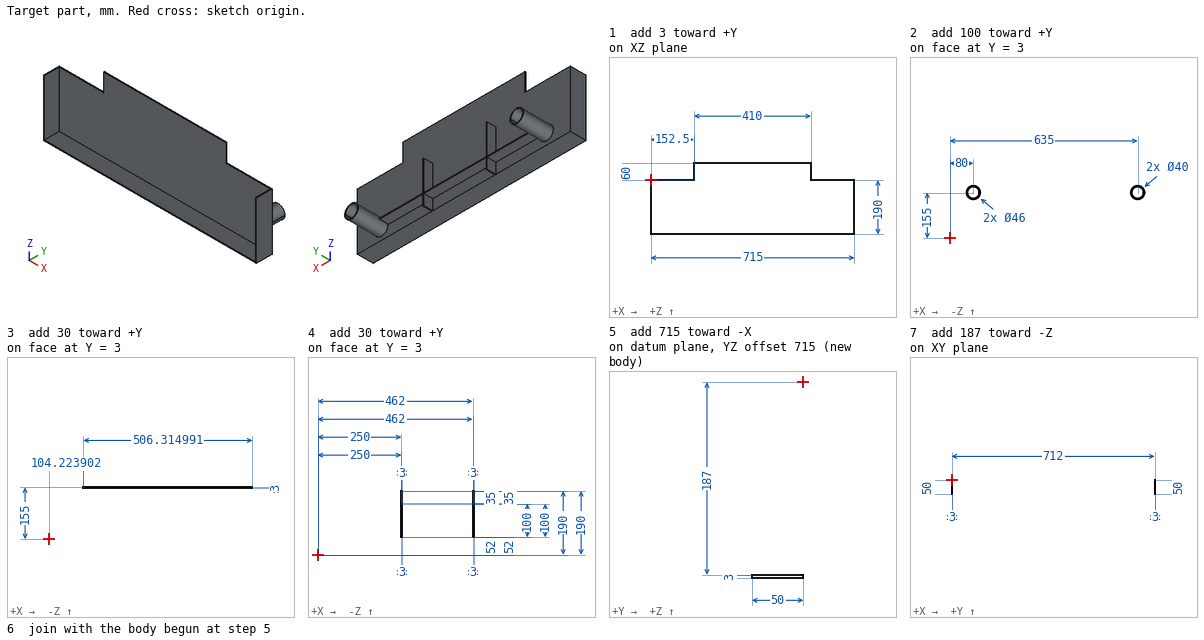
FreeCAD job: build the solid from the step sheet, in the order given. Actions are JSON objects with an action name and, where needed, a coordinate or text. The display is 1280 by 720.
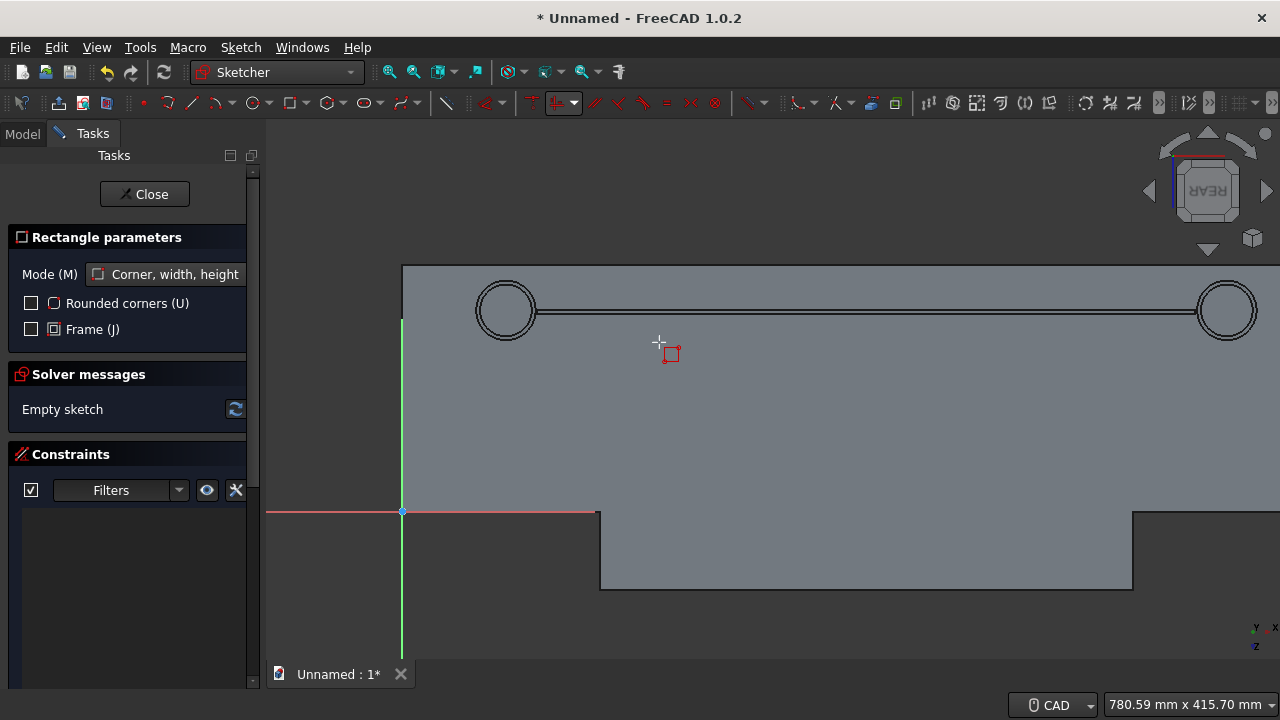
{"action": "scroll", "coordinate": [727, 265], "scroll_direction": "up", "scroll_amount": 8}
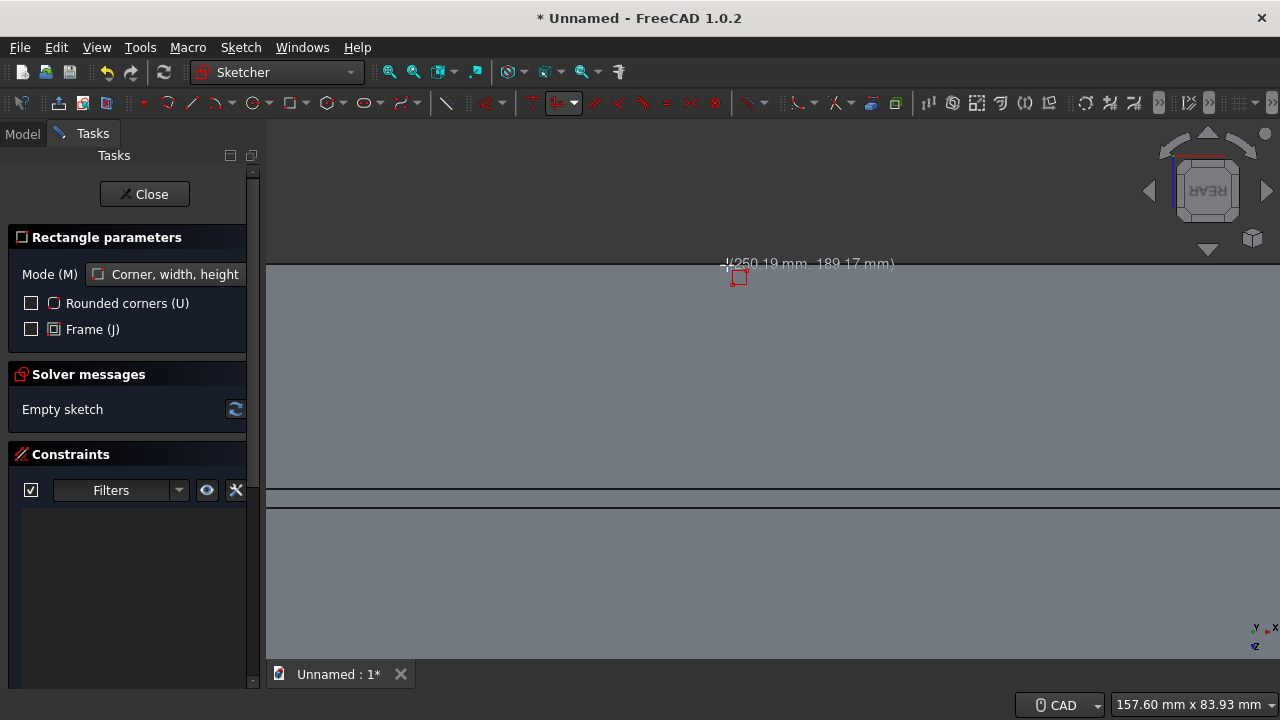
{"action": "scroll", "coordinate": [728, 266], "scroll_direction": "down", "scroll_amount": 8}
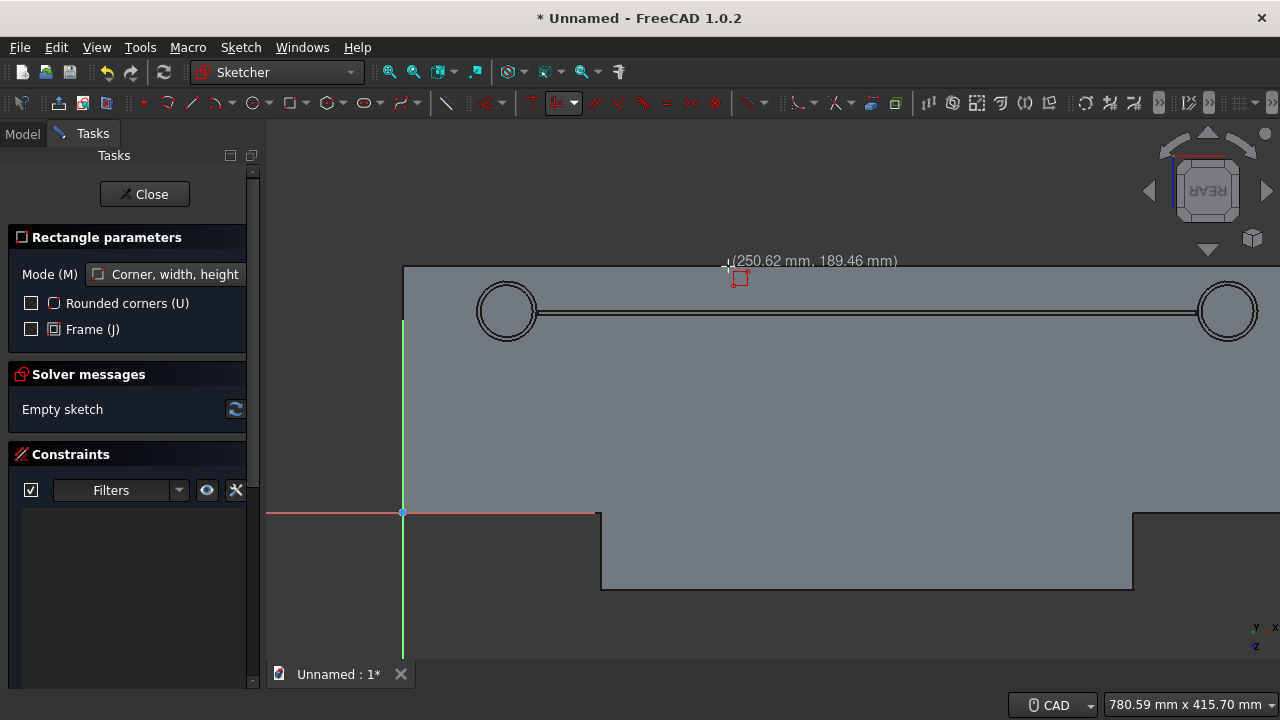
{"action": "left_click", "coordinate": [728, 266]}
{"action": "mouse_move", "coordinate": [731, 311]}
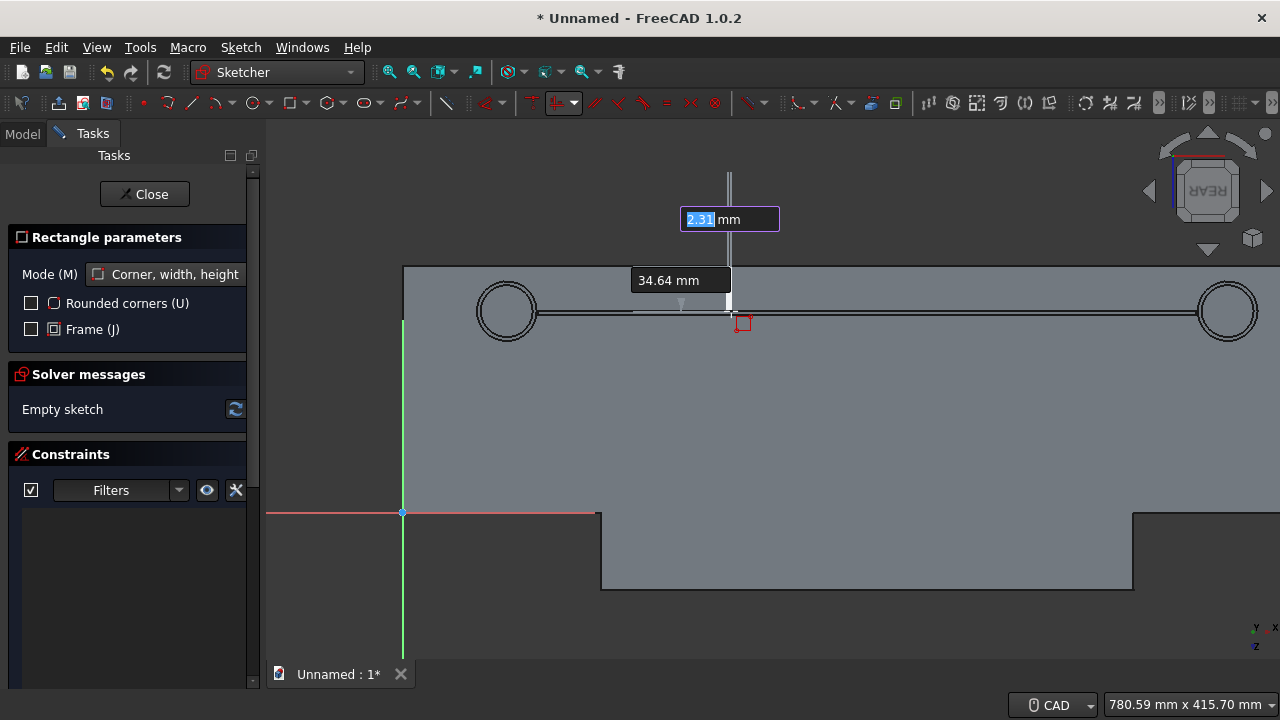
{"action": "type", "text": "3"}
{"action": "key", "text": "Tab"}
{"action": "type", "text": "35"}
{"action": "key", "text": "Return"}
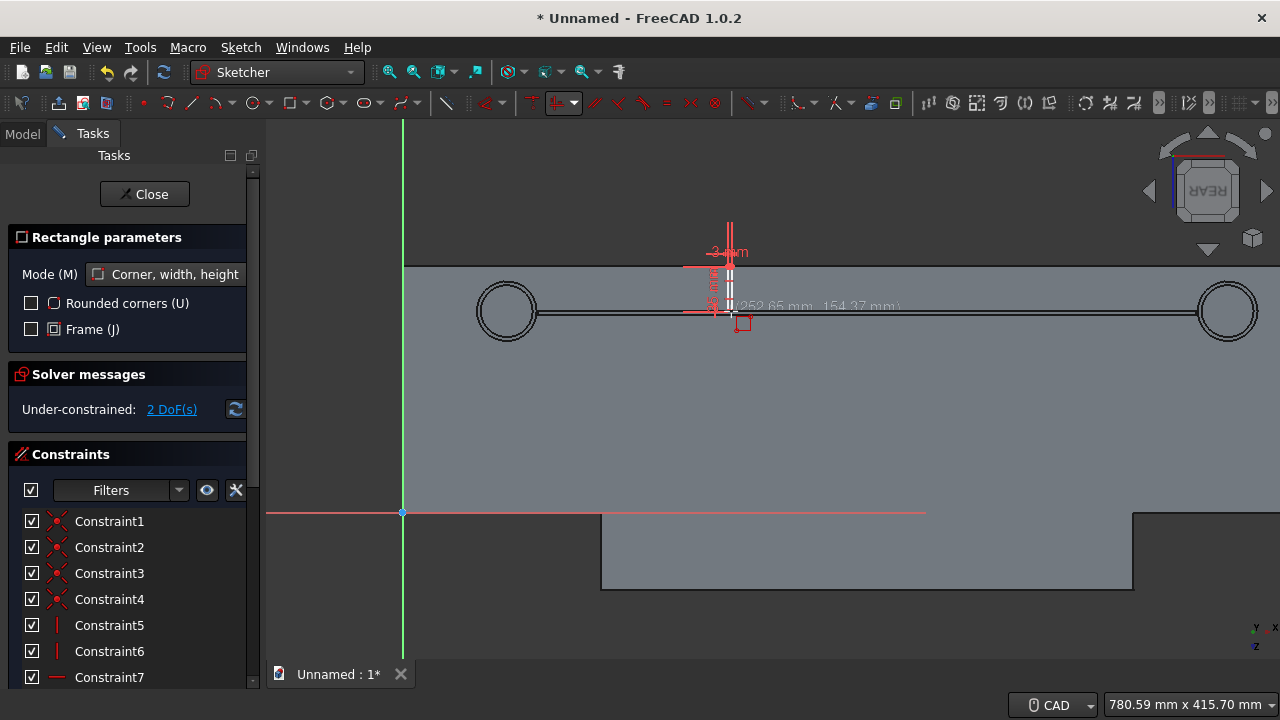
{"action": "scroll", "coordinate": [728, 315], "scroll_direction": "up", "scroll_amount": 8}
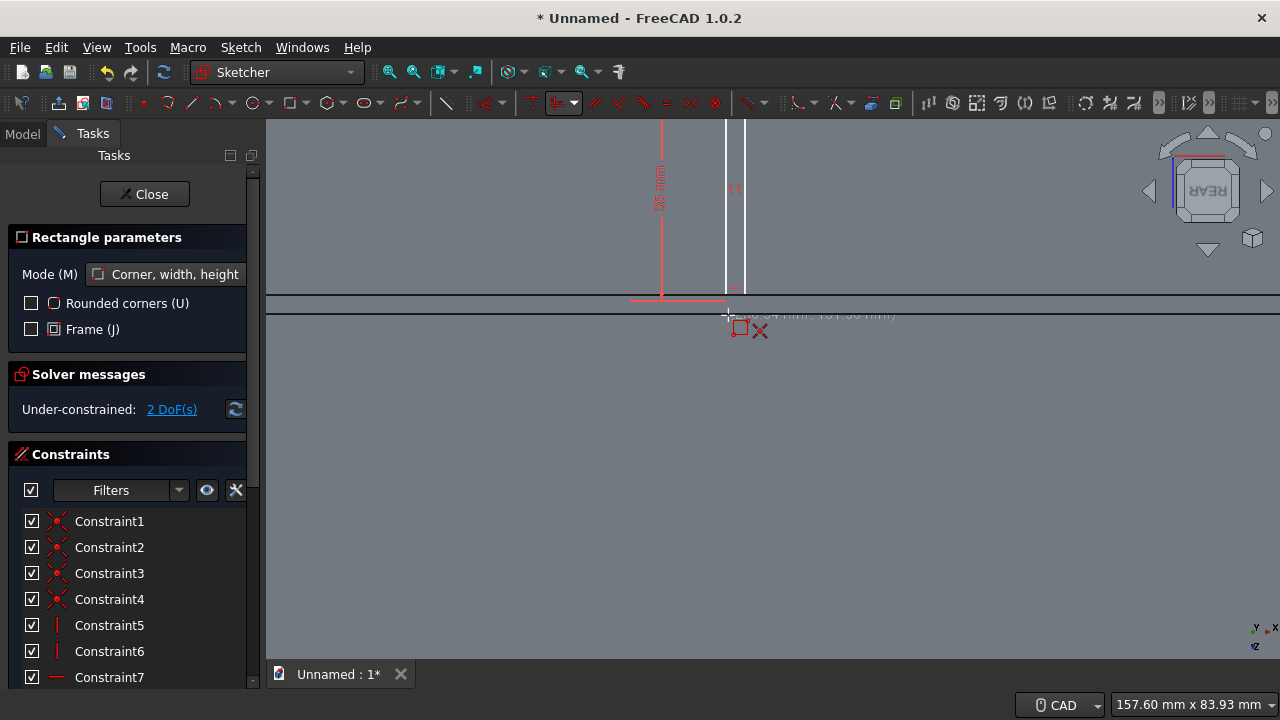
{"action": "left_click", "coordinate": [724, 314]}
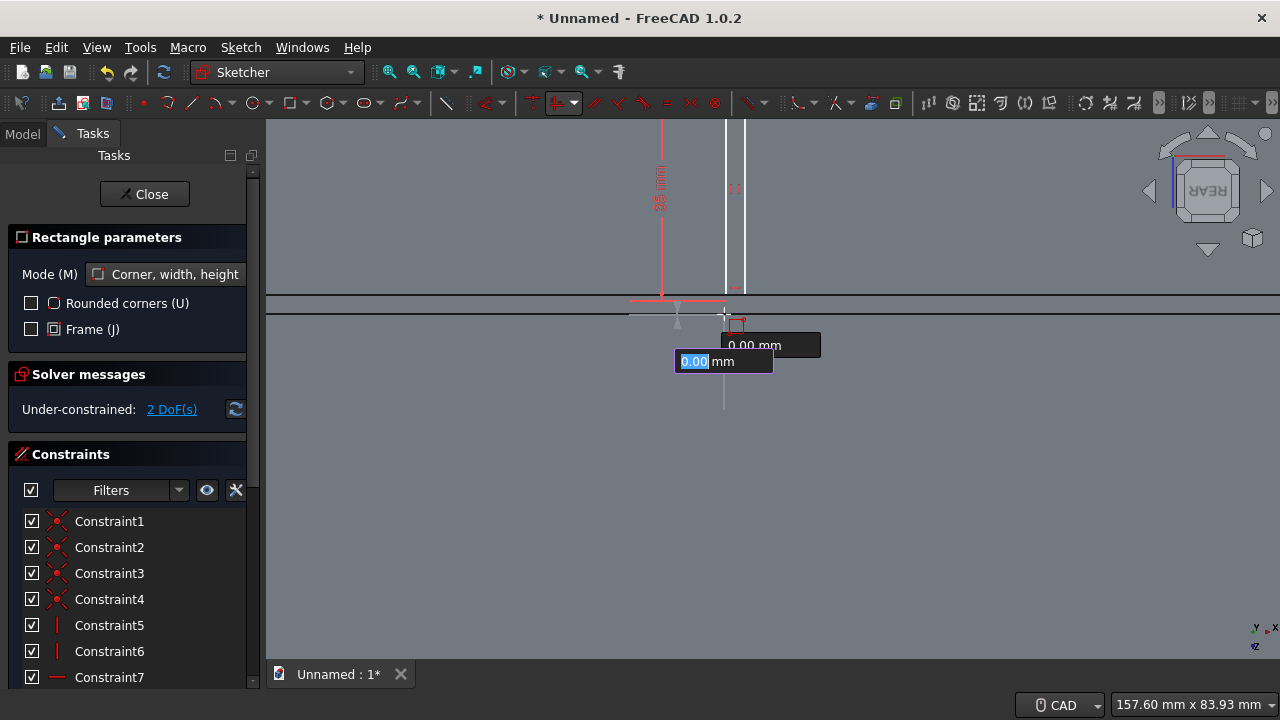
{"action": "scroll", "coordinate": [728, 315], "scroll_direction": "down", "scroll_amount": 8}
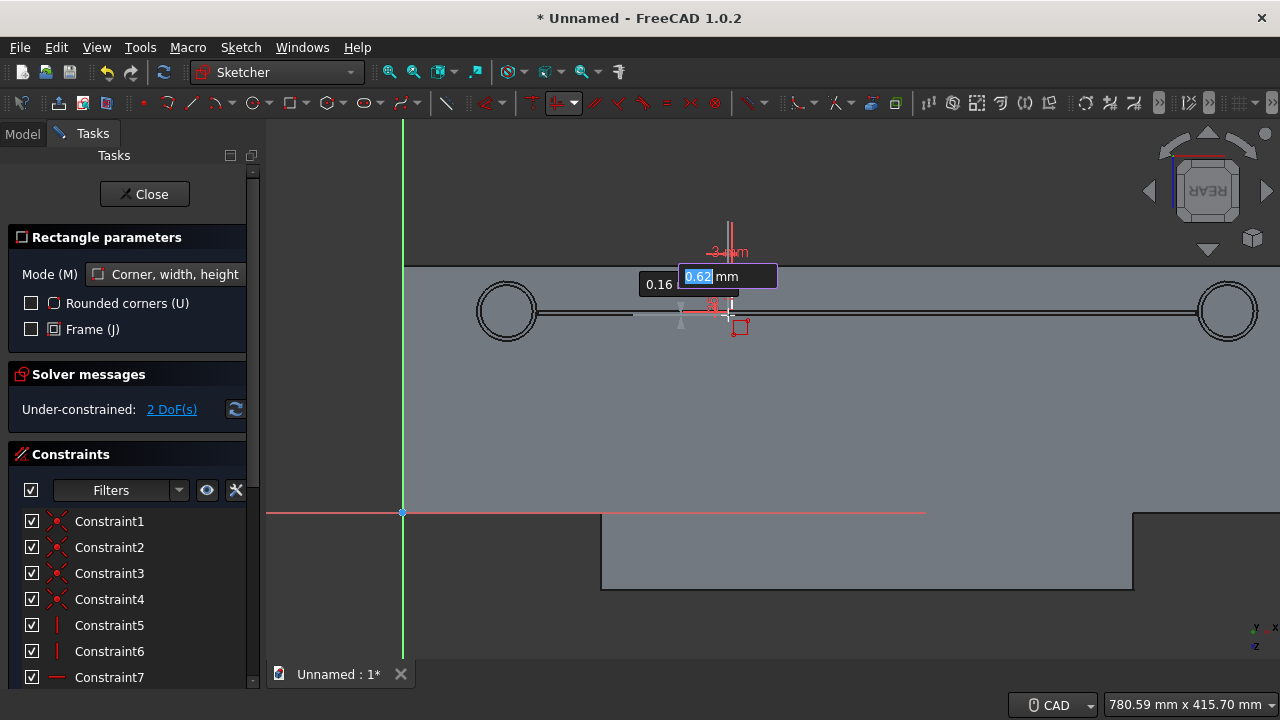
{"action": "left_click", "coordinate": [731, 445]}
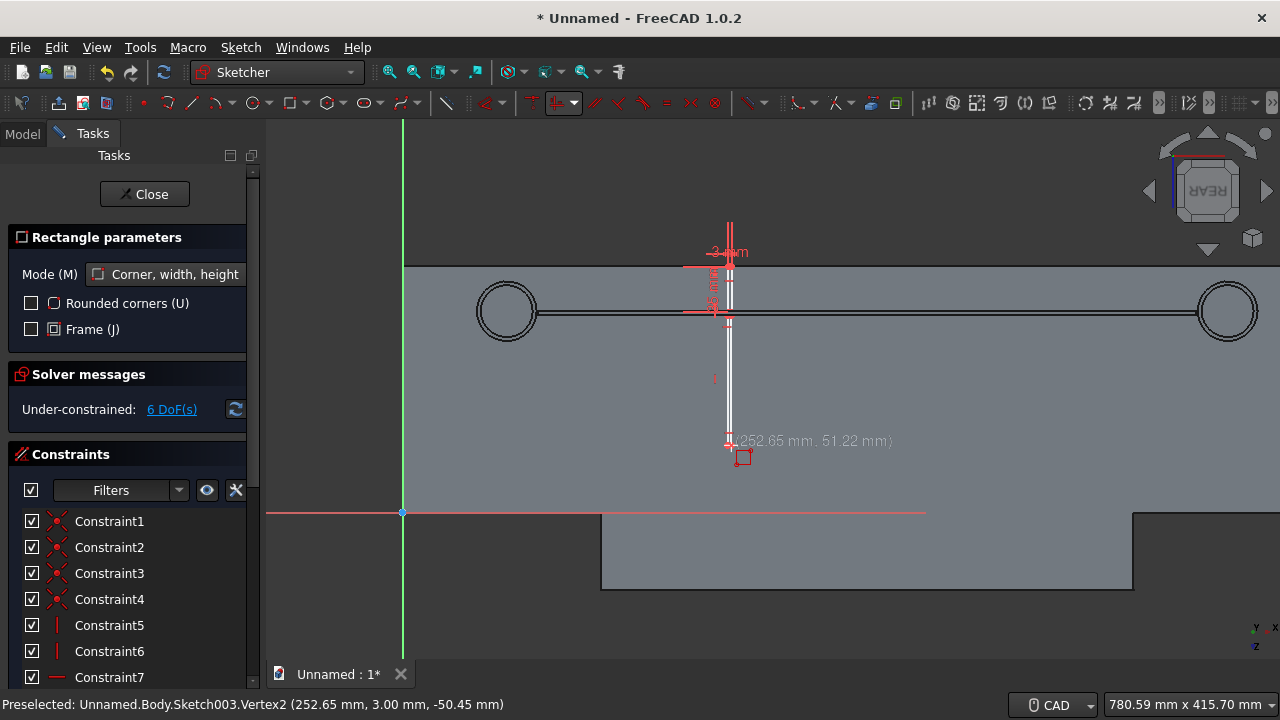
{"action": "scroll", "coordinate": [1003, 315], "scroll_direction": "up", "scroll_amount": 8}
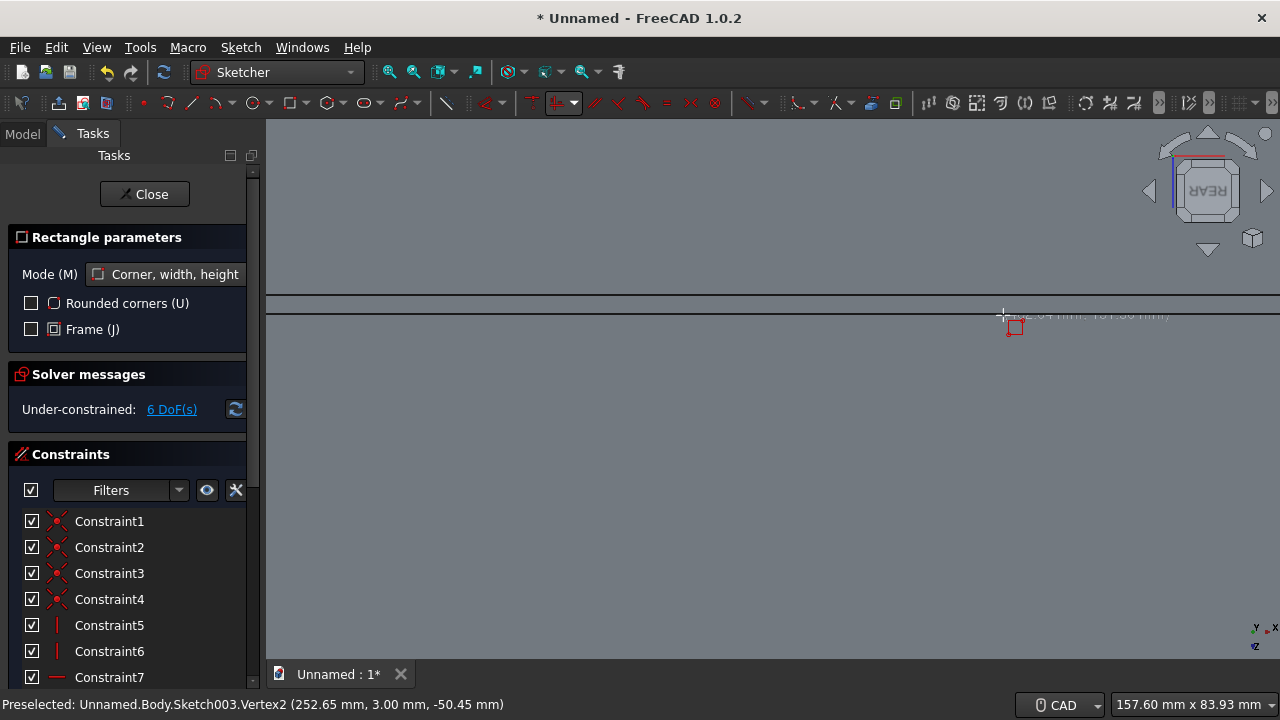
{"action": "scroll", "coordinate": [1003, 315], "scroll_direction": "down", "scroll_amount": 8}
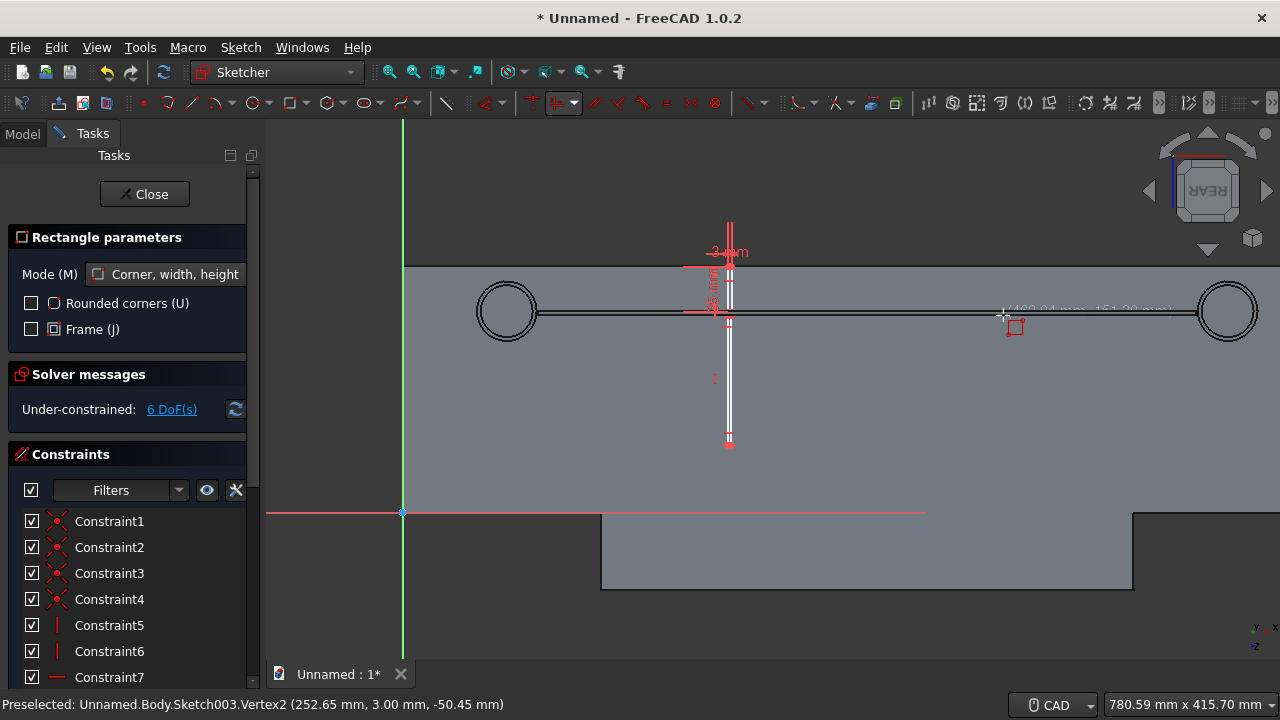
{"action": "left_click", "coordinate": [1003, 315]}
{"action": "mouse_move", "coordinate": [1007, 445]}